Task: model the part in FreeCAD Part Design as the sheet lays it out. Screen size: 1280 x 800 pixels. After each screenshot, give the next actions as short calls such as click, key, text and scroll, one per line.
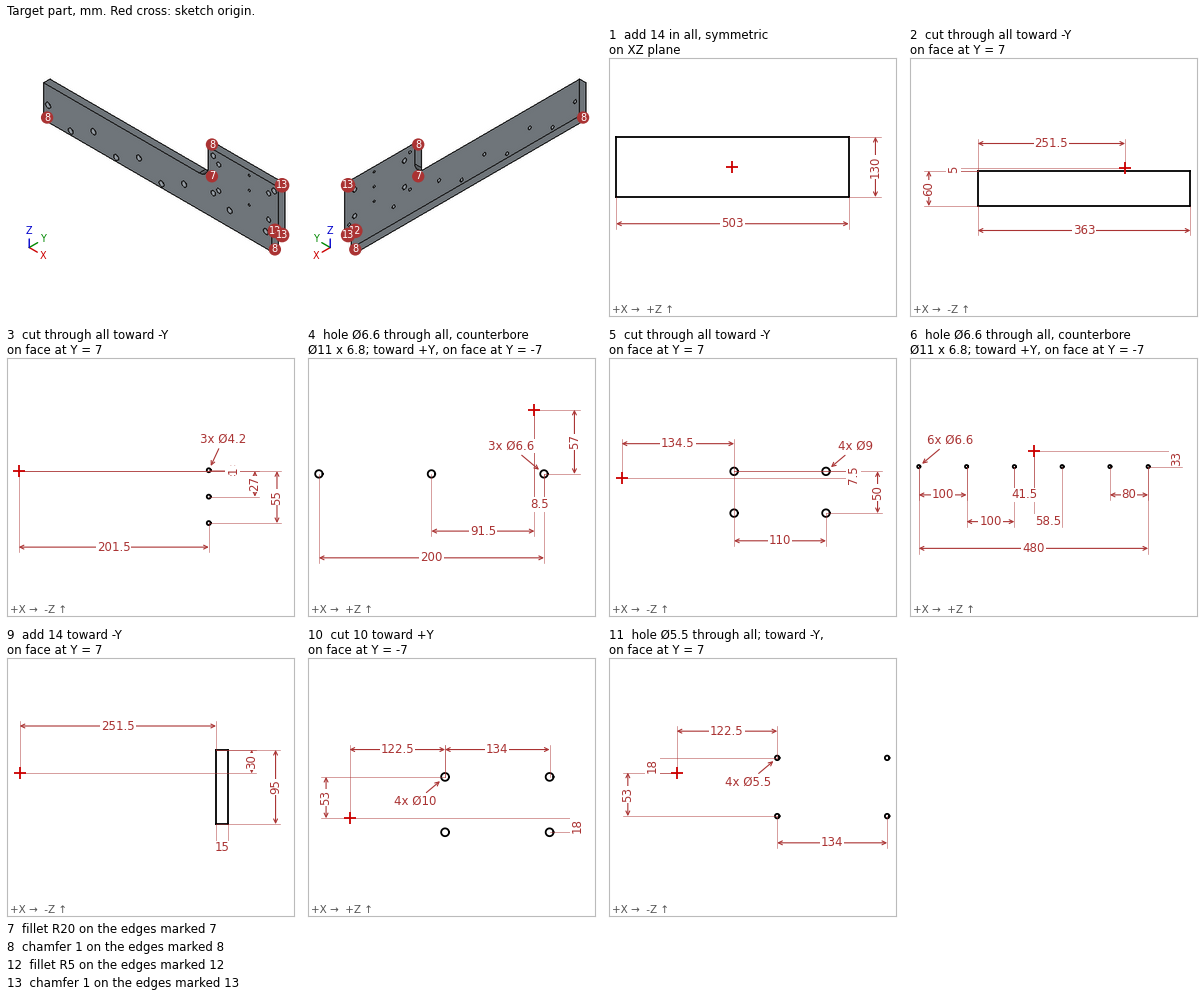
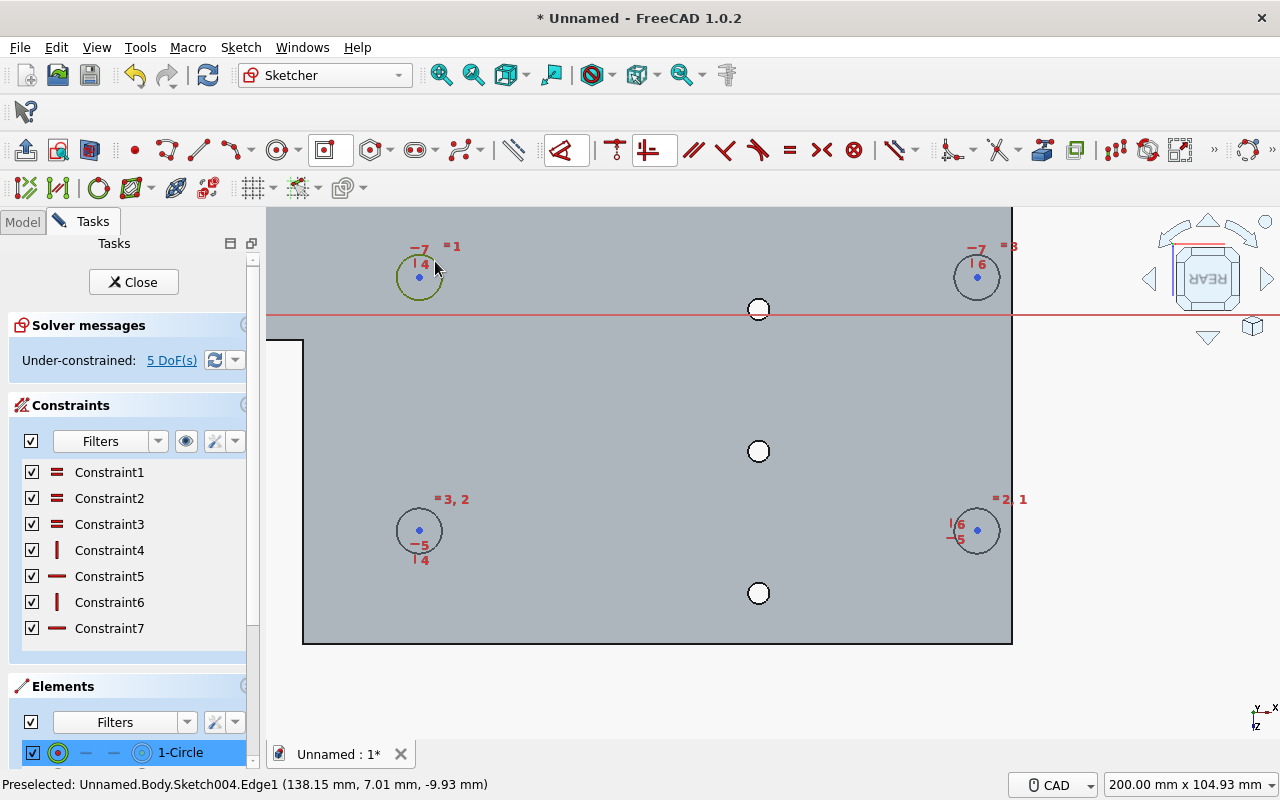
key(k)
key(o)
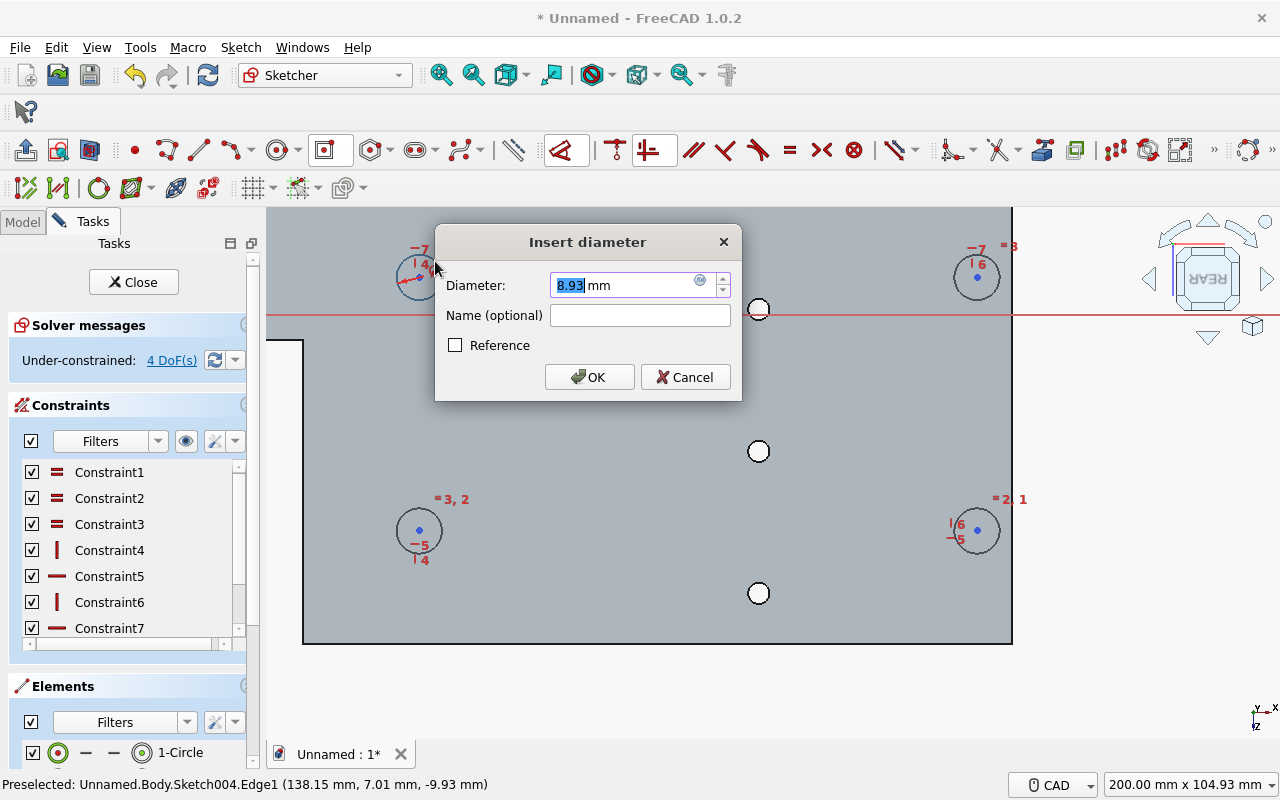
text(9)
key(Return)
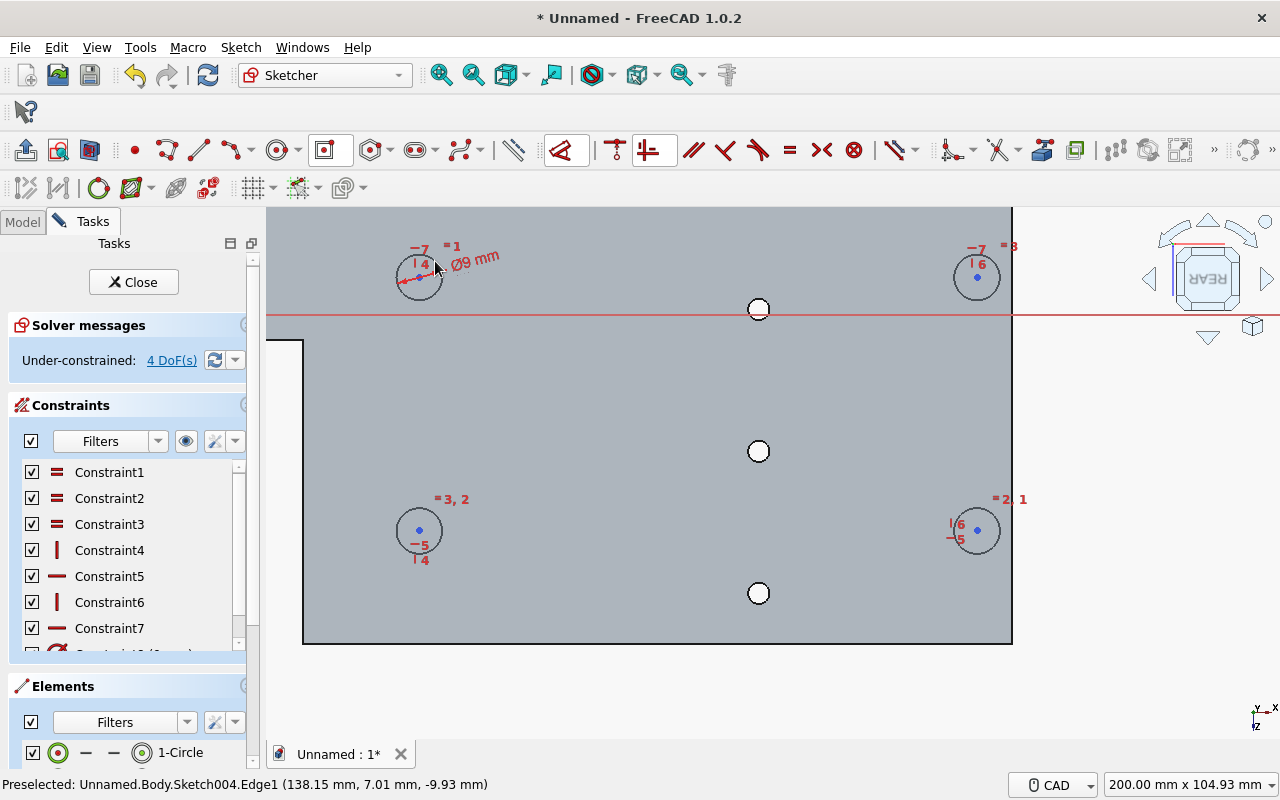
click(419, 277)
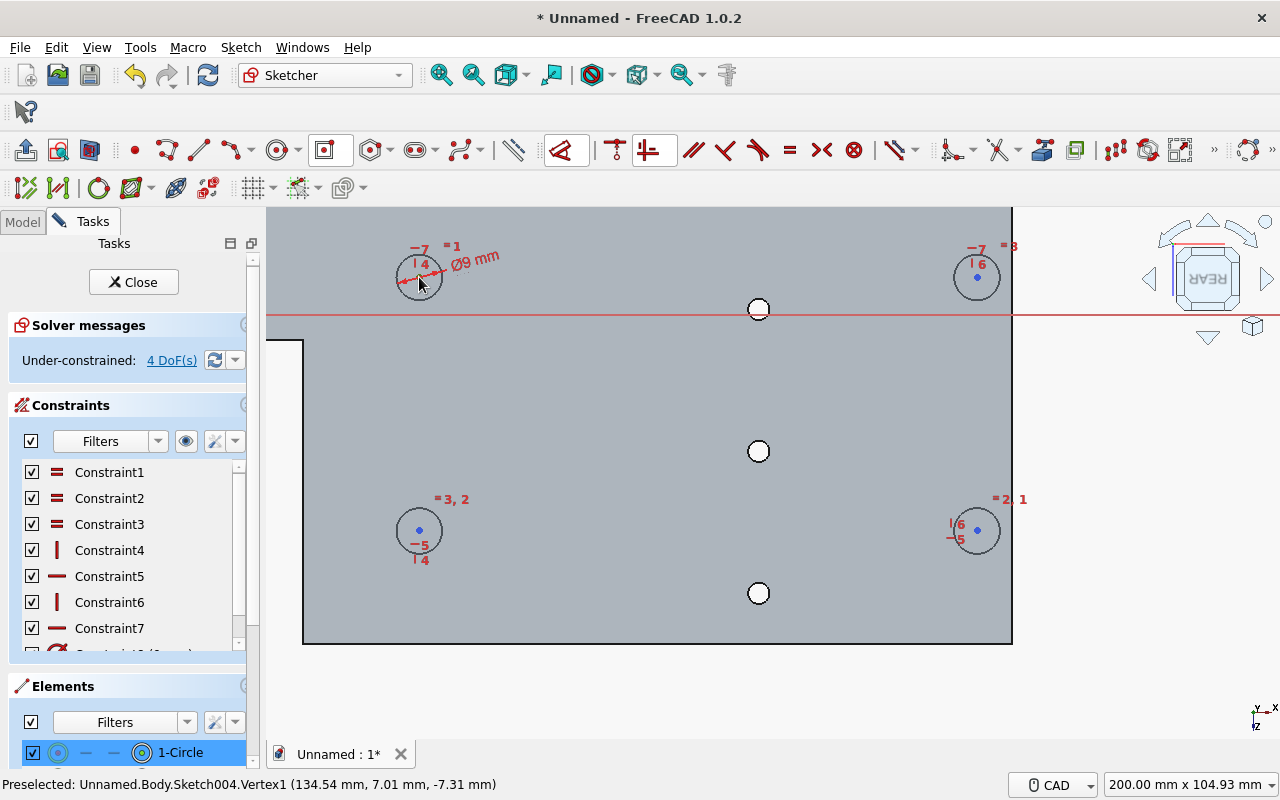
key(i)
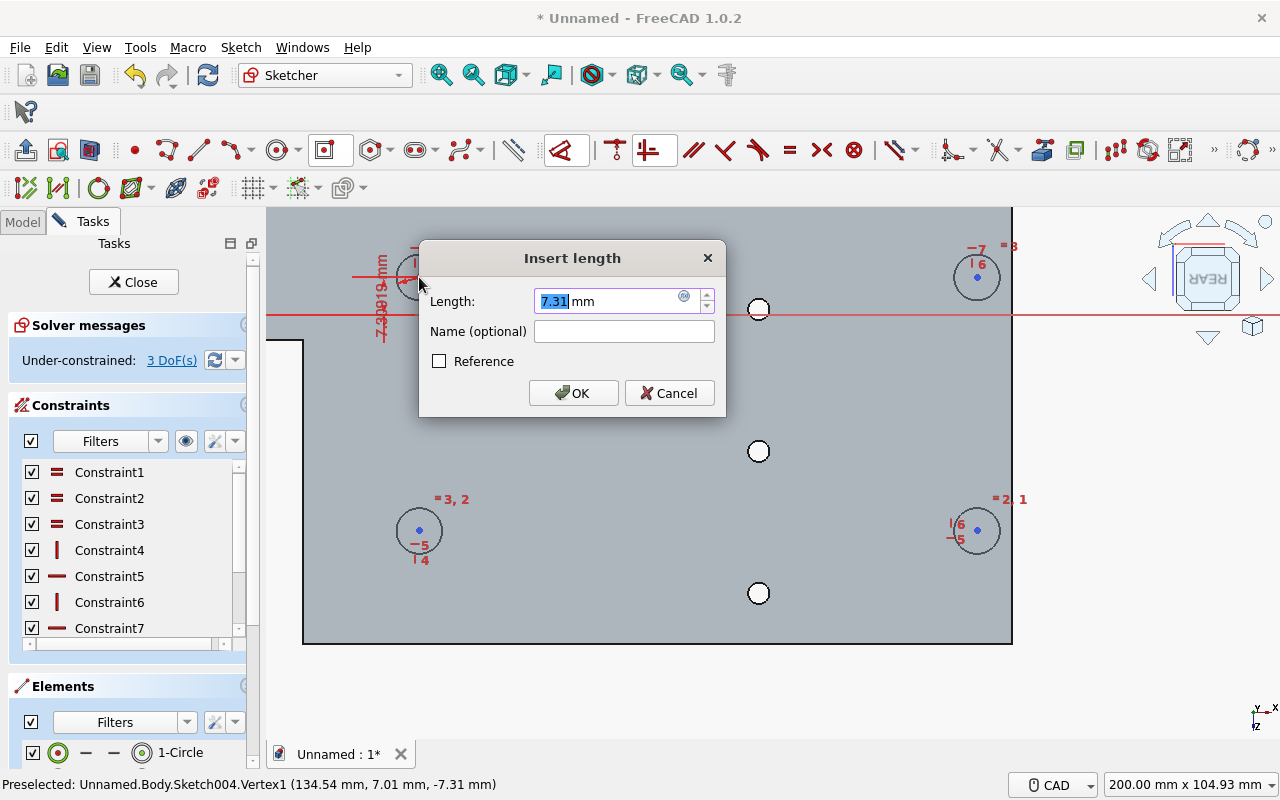
text(7.5)
key(Return)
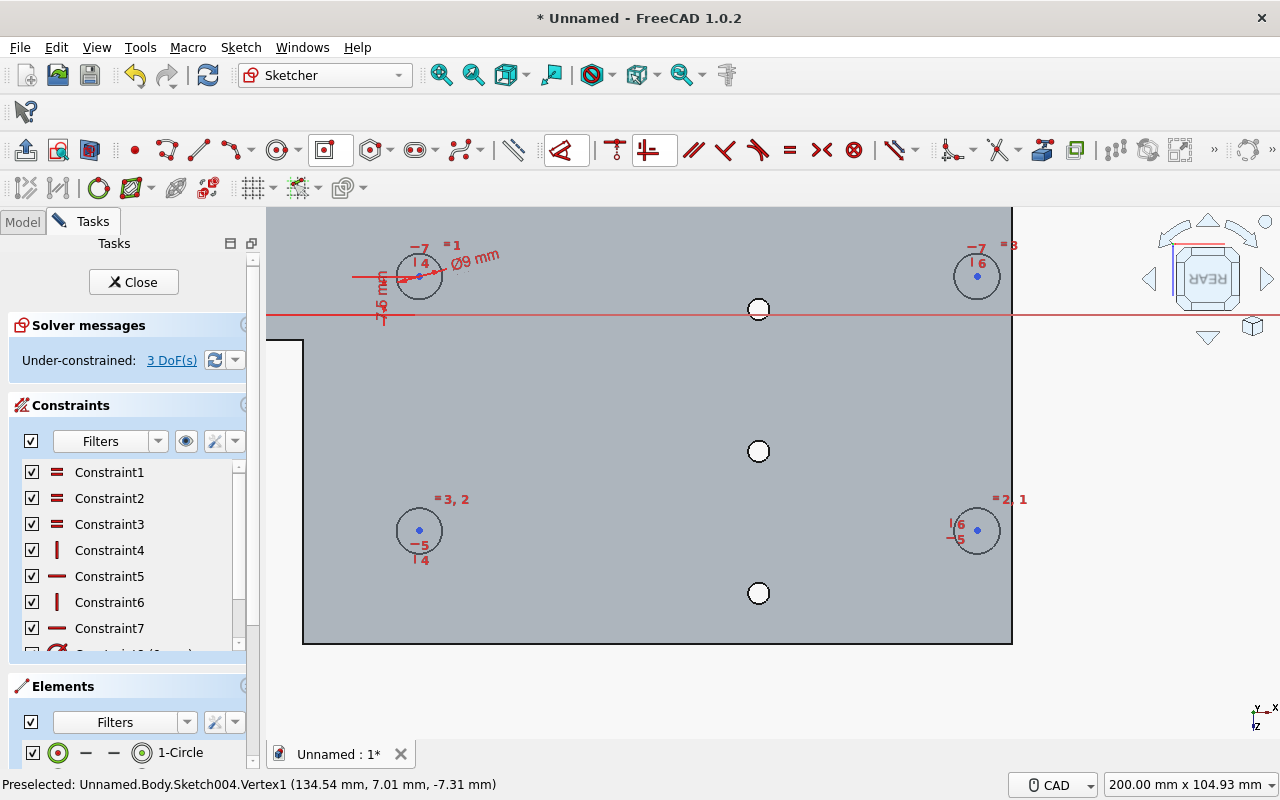
click(419, 277)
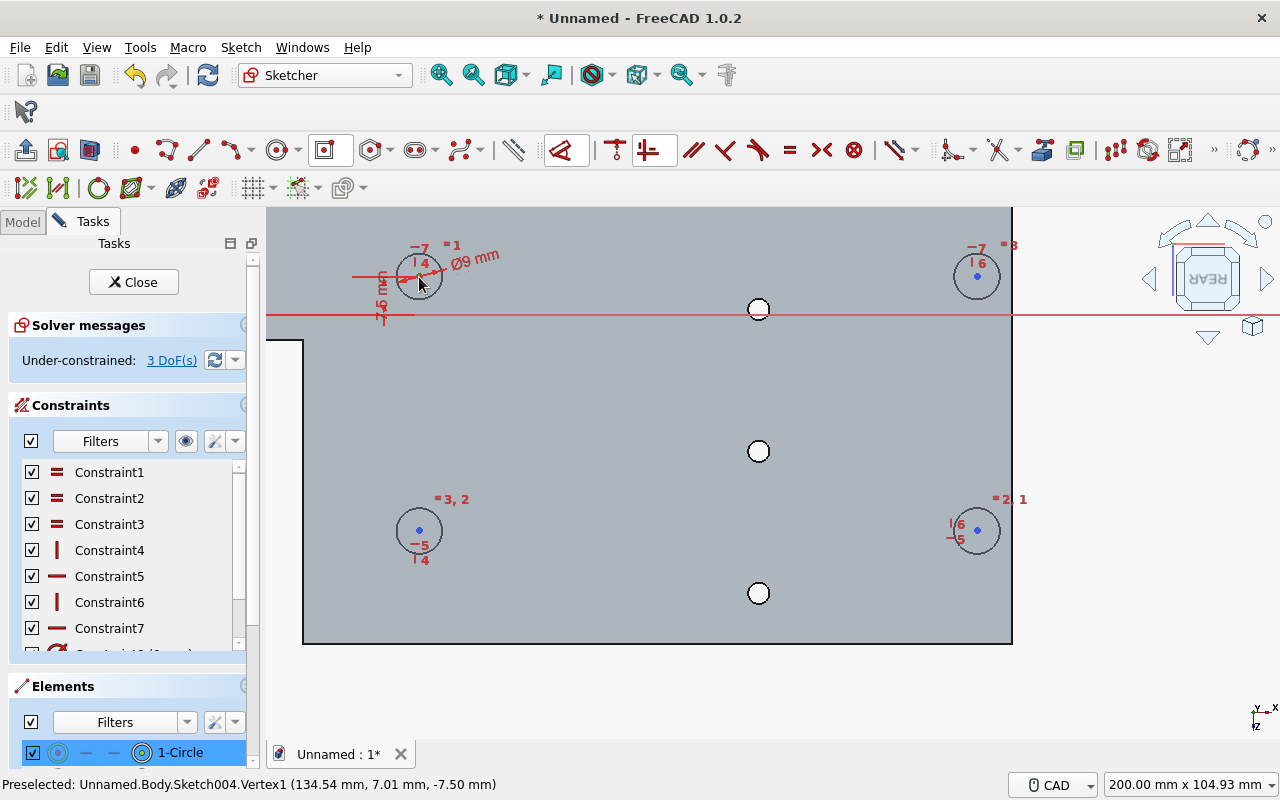
click(977, 531)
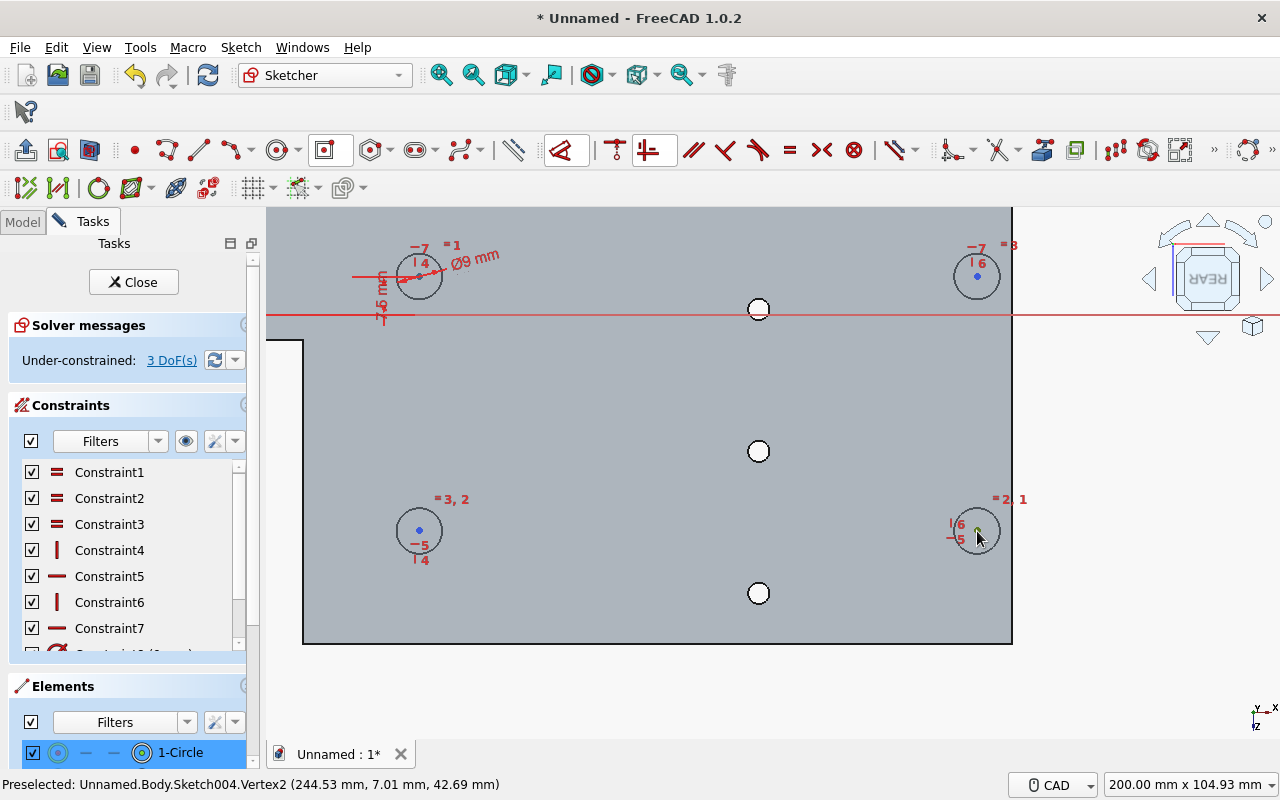
key(i)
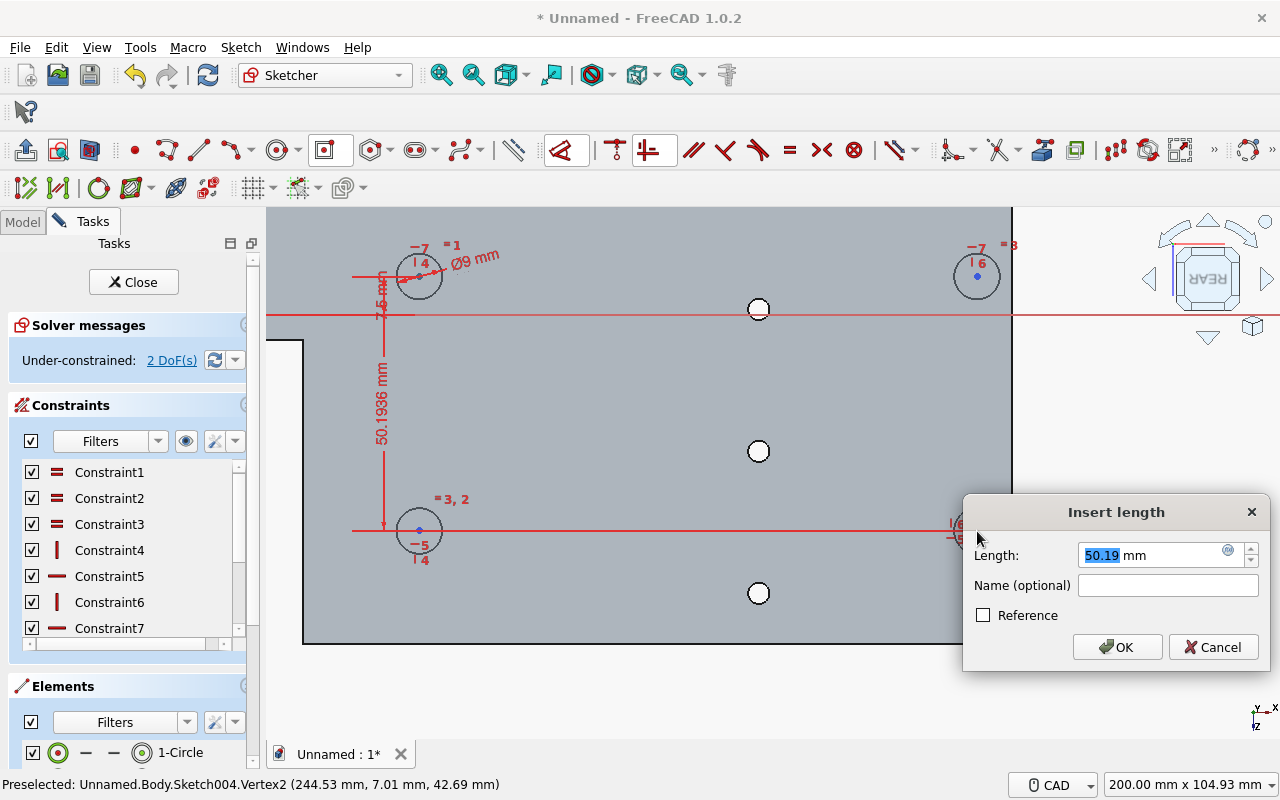
text(50)
key(Return)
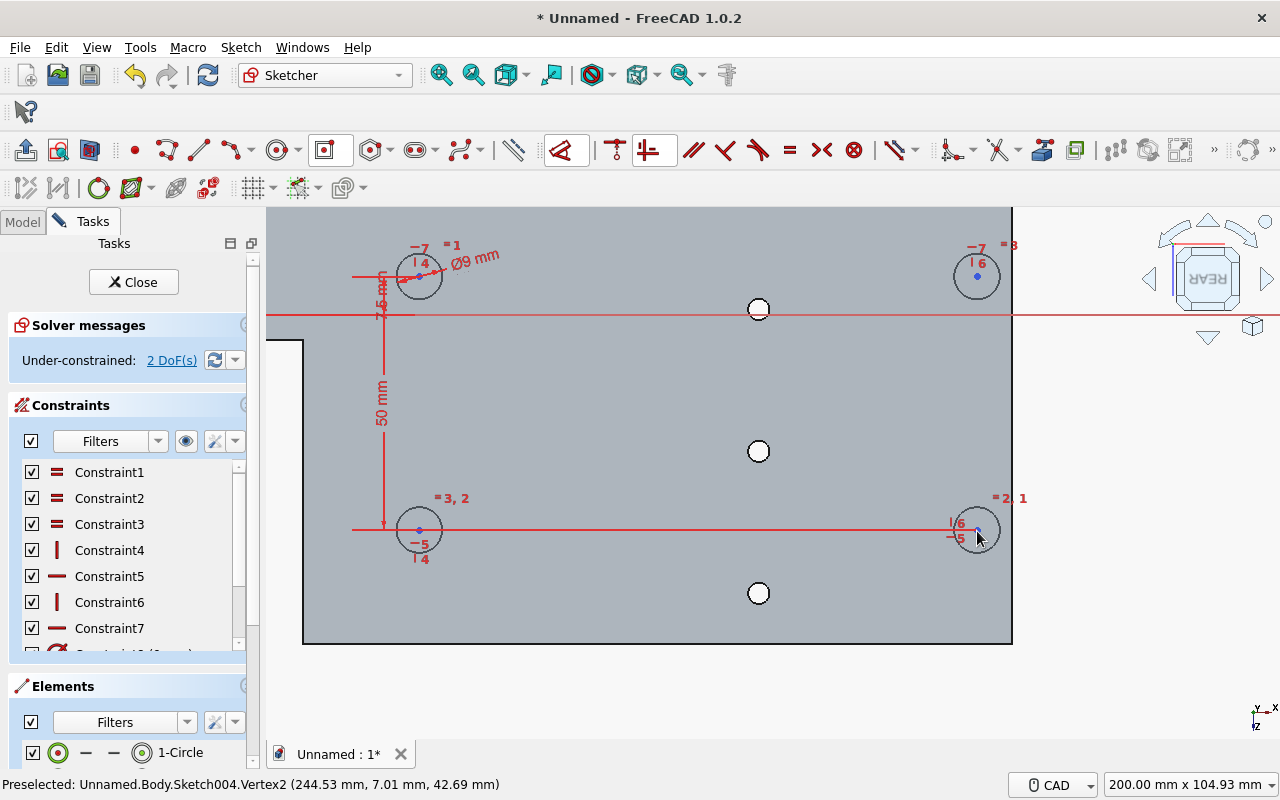
click(419, 277)